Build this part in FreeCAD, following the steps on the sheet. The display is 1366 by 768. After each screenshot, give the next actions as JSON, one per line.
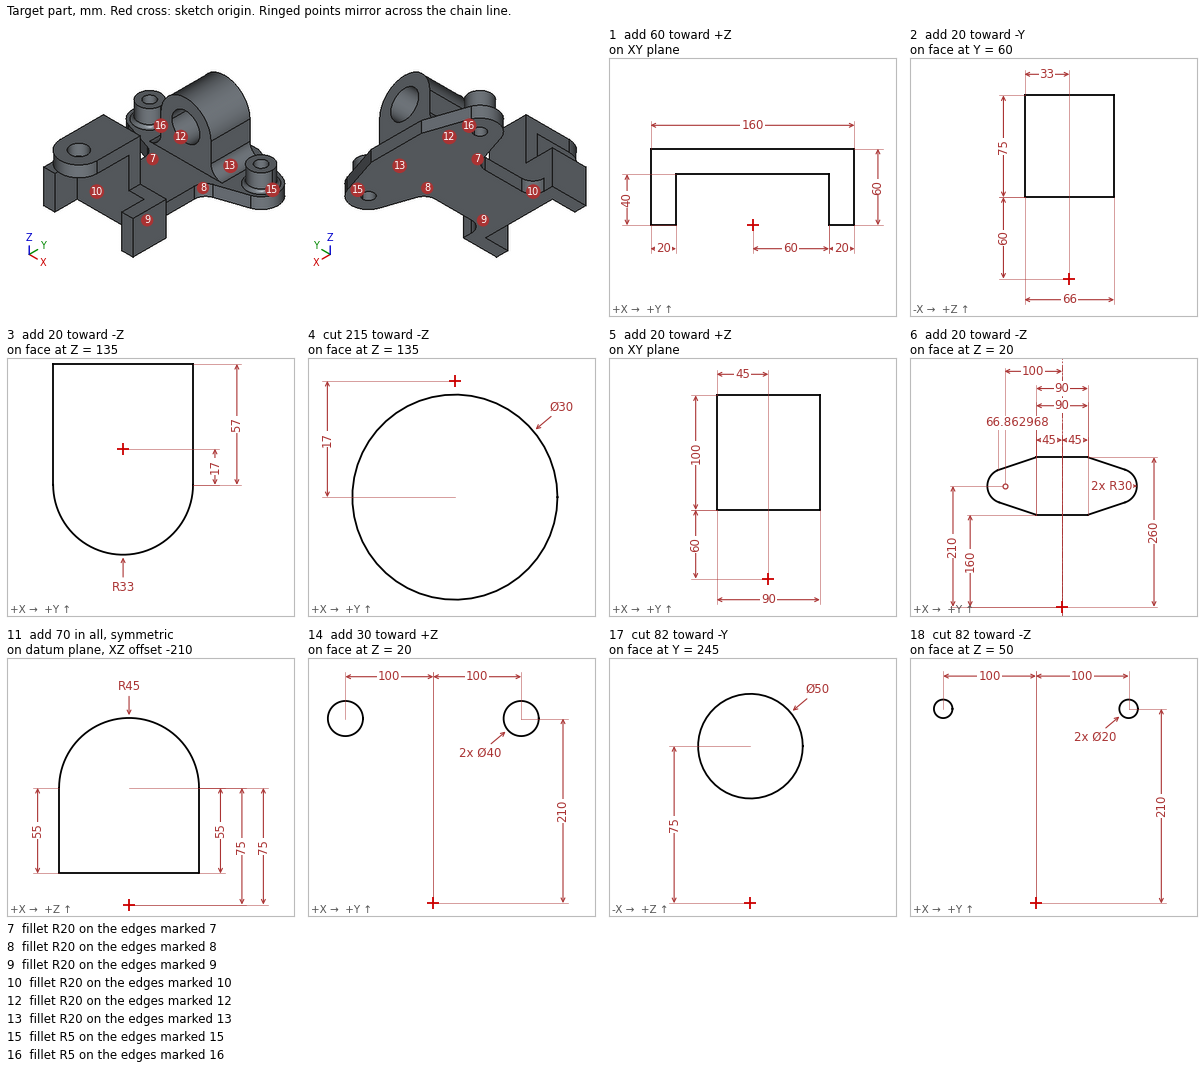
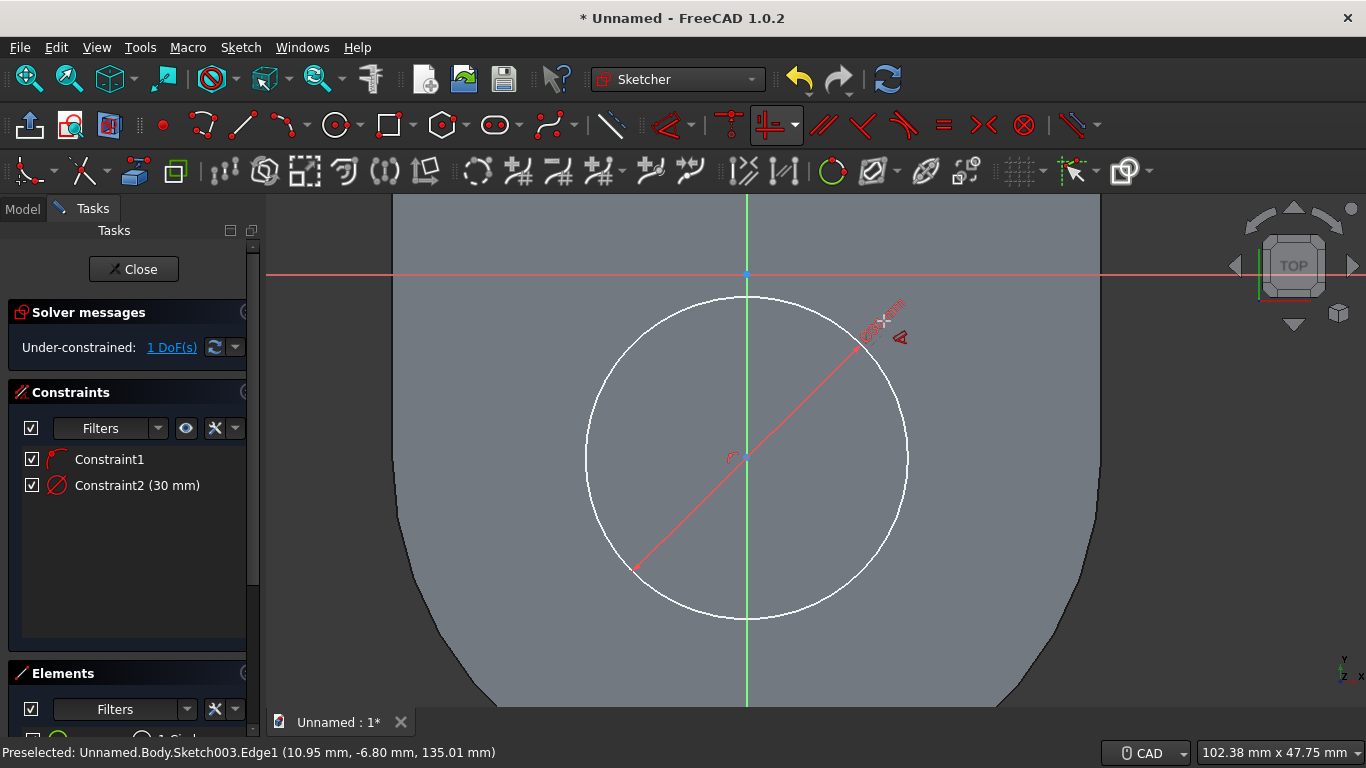
{"action": "left_click", "coordinate": [747, 458]}
{"action": "left_click", "coordinate": [781, 366]}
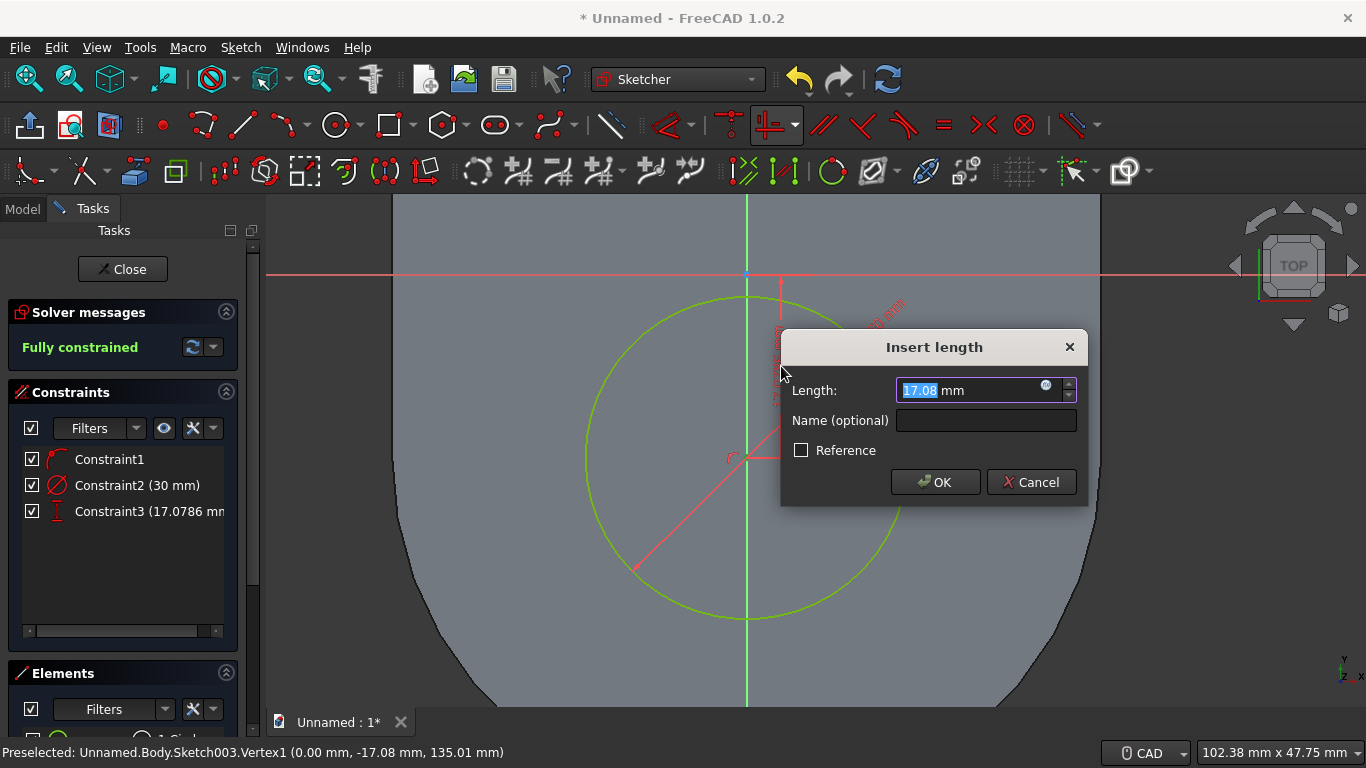
{"action": "type", "text": "17"}
{"action": "key", "text": "Return"}
{"action": "key", "text": "Escape"}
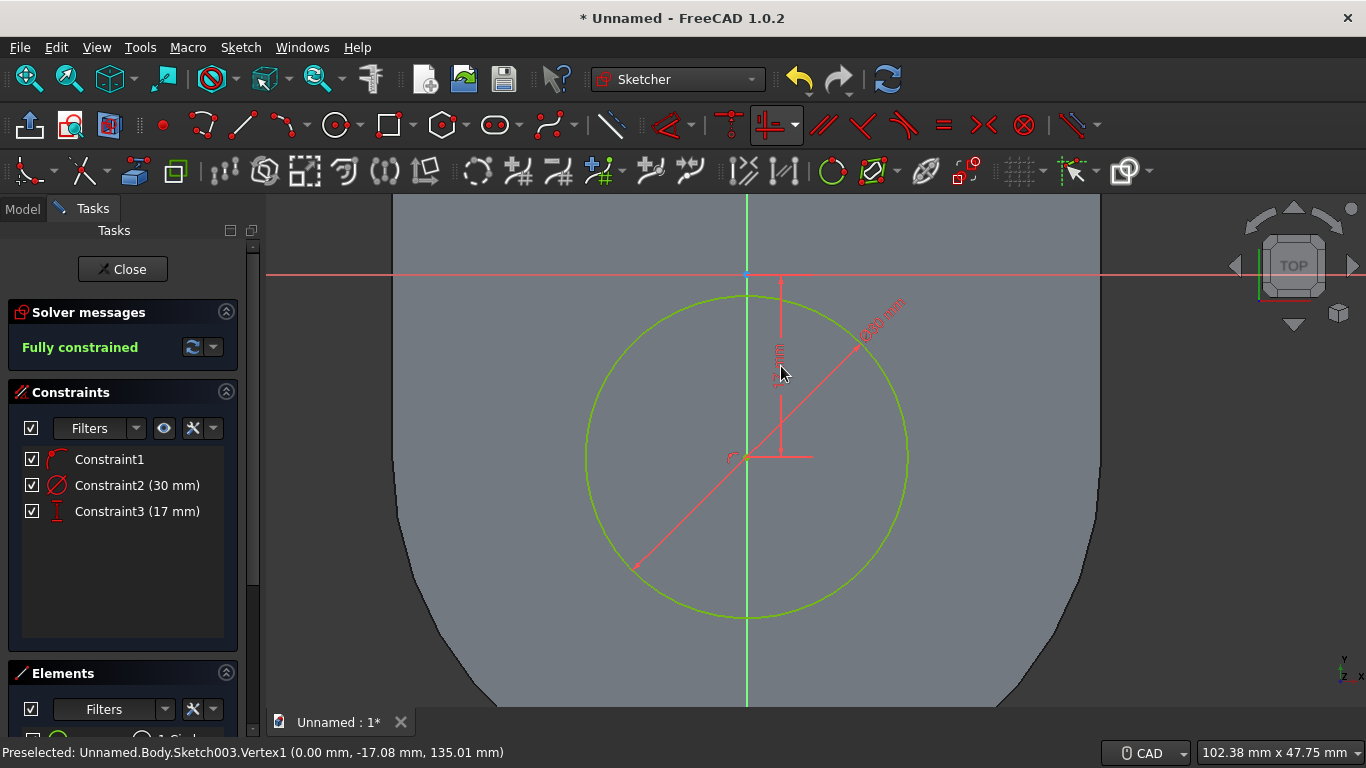
{"action": "left_click", "coordinate": [123, 269]}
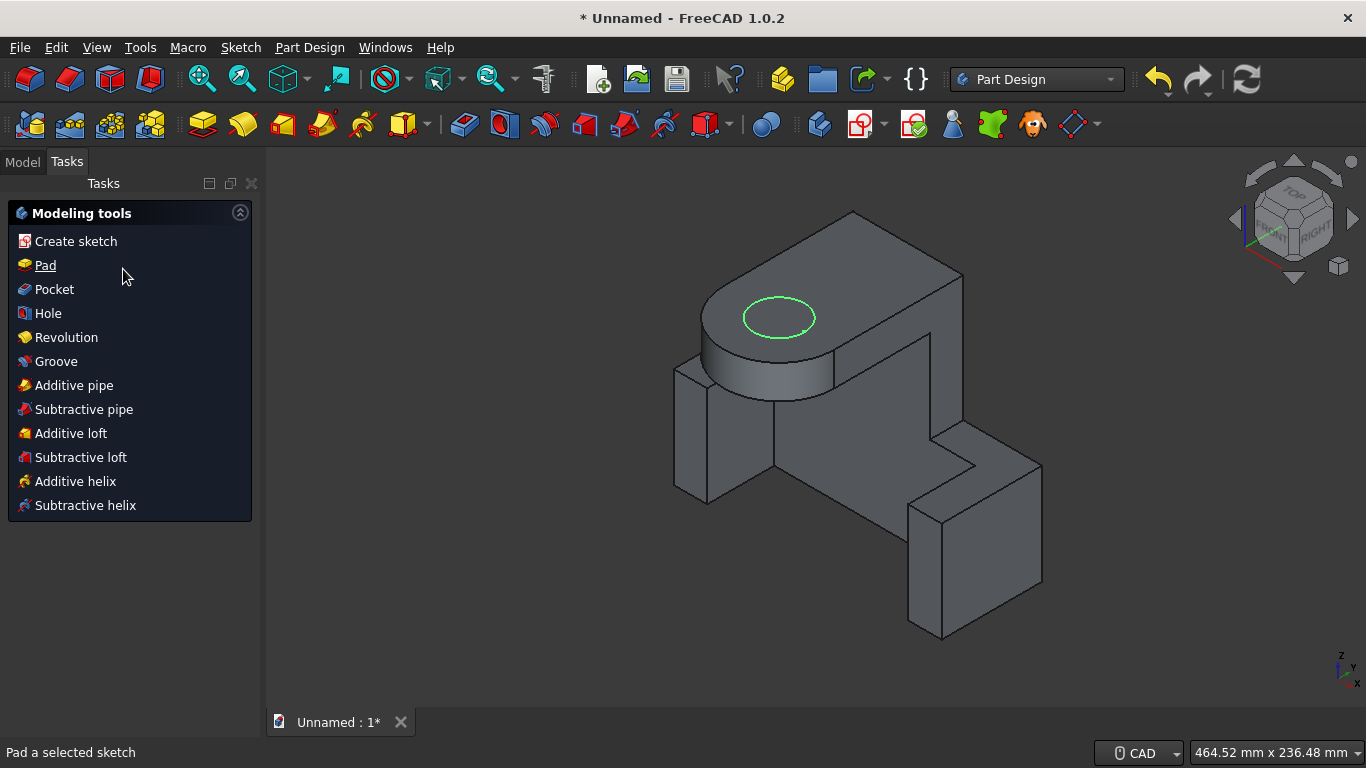
{"action": "left_click", "coordinate": [466, 124]}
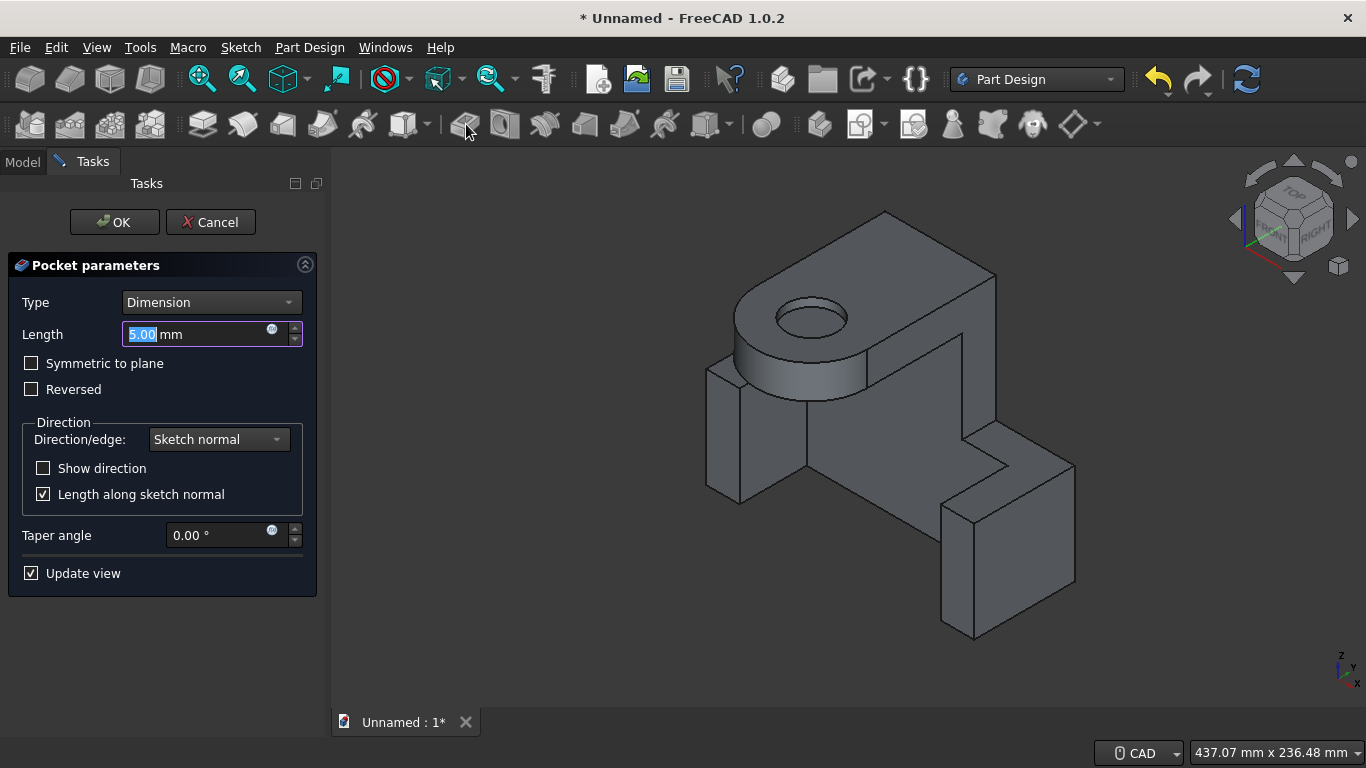
{"action": "type", "text": "215"}
{"action": "key", "text": "Tab"}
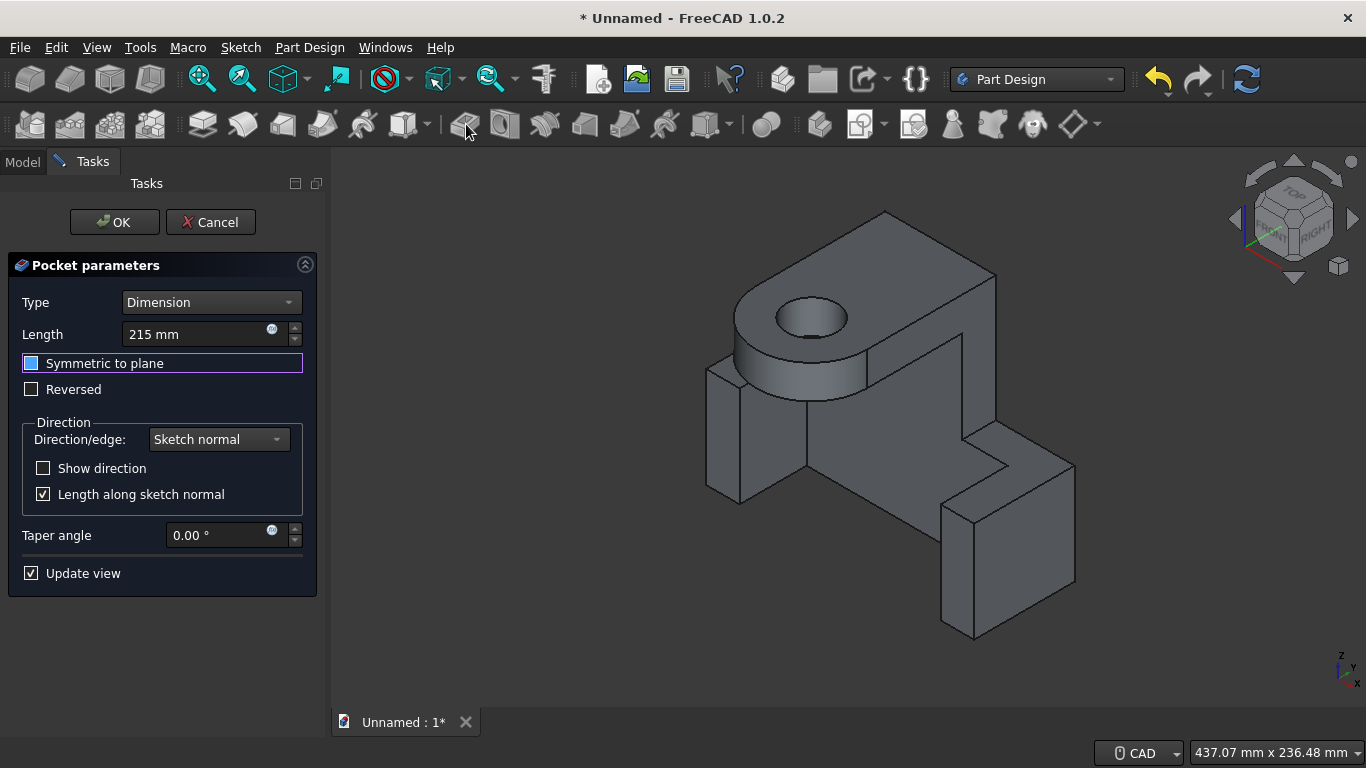
{"action": "left_click", "coordinate": [115, 222]}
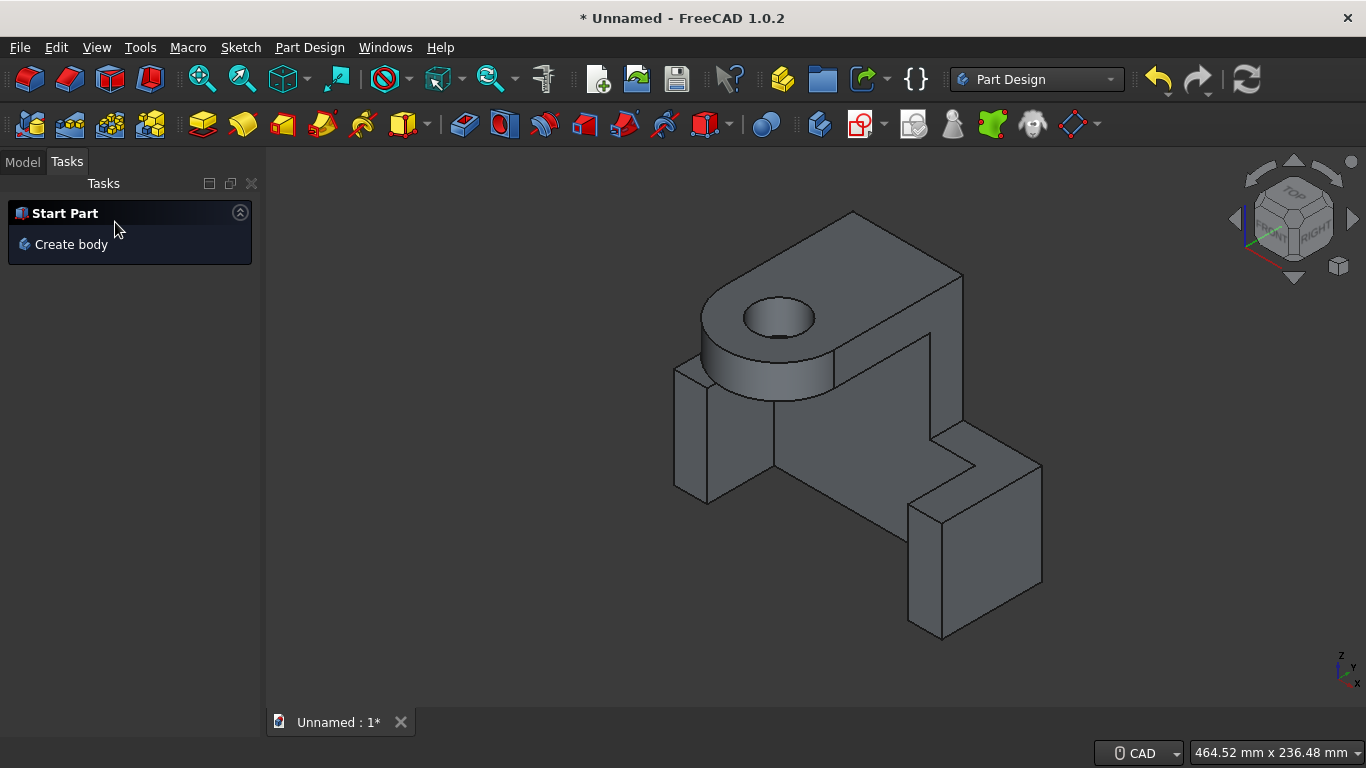
{"action": "left_click", "coordinate": [860, 124]}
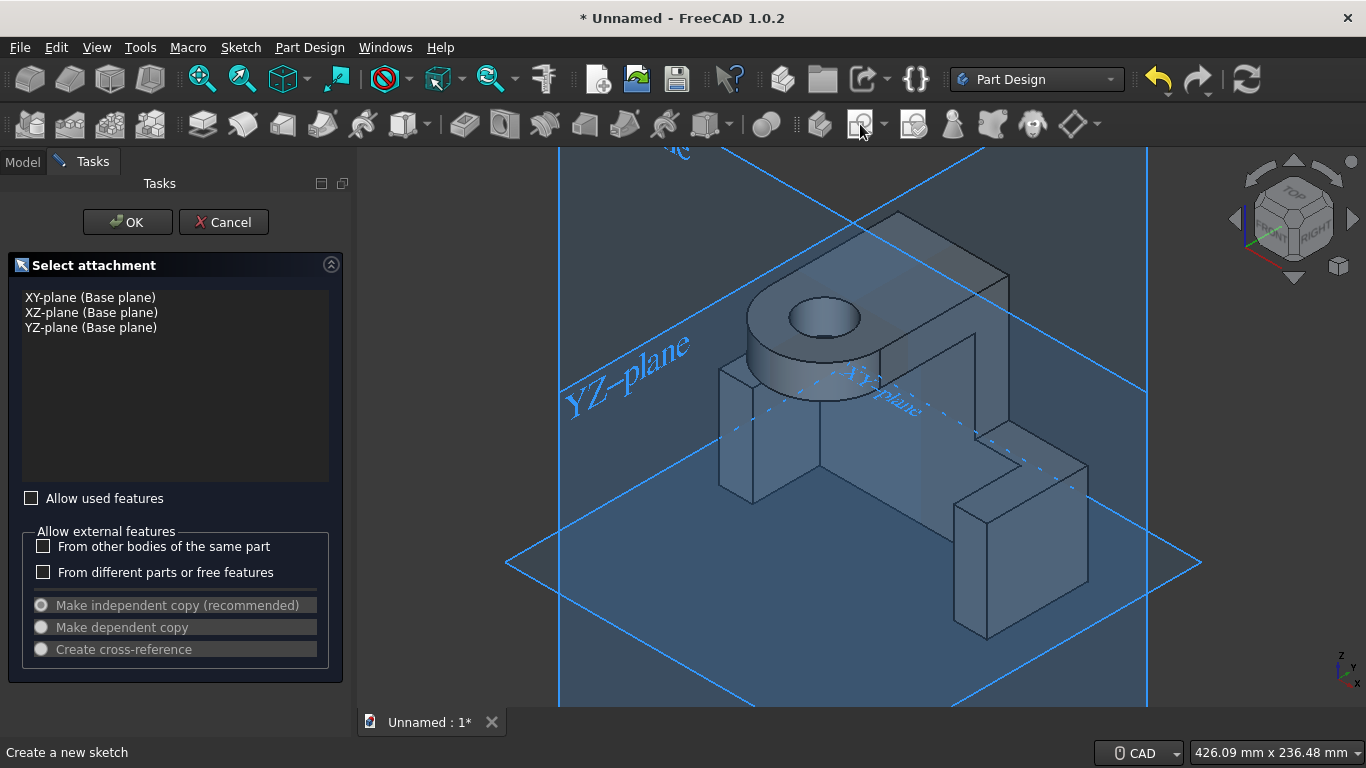
{"action": "left_click", "coordinate": [82, 298]}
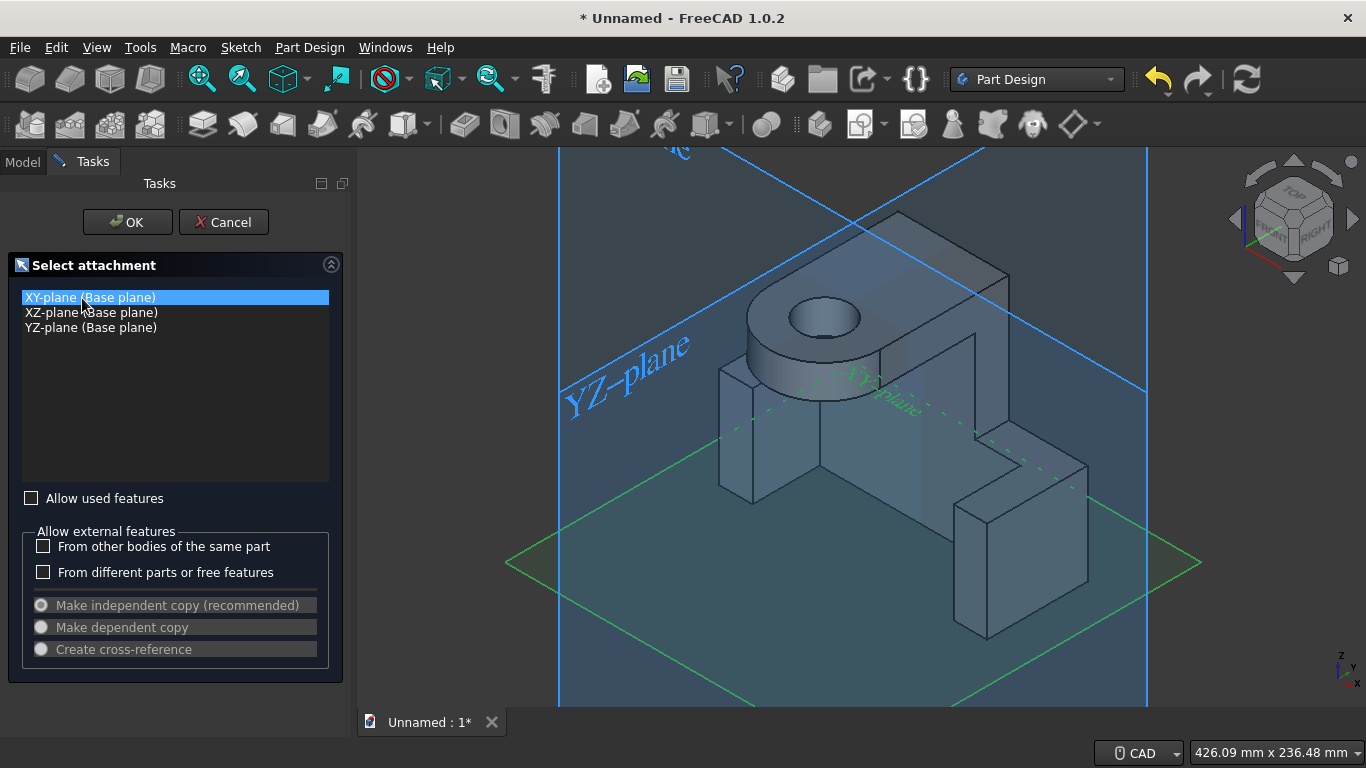
{"action": "left_click", "coordinate": [128, 222]}